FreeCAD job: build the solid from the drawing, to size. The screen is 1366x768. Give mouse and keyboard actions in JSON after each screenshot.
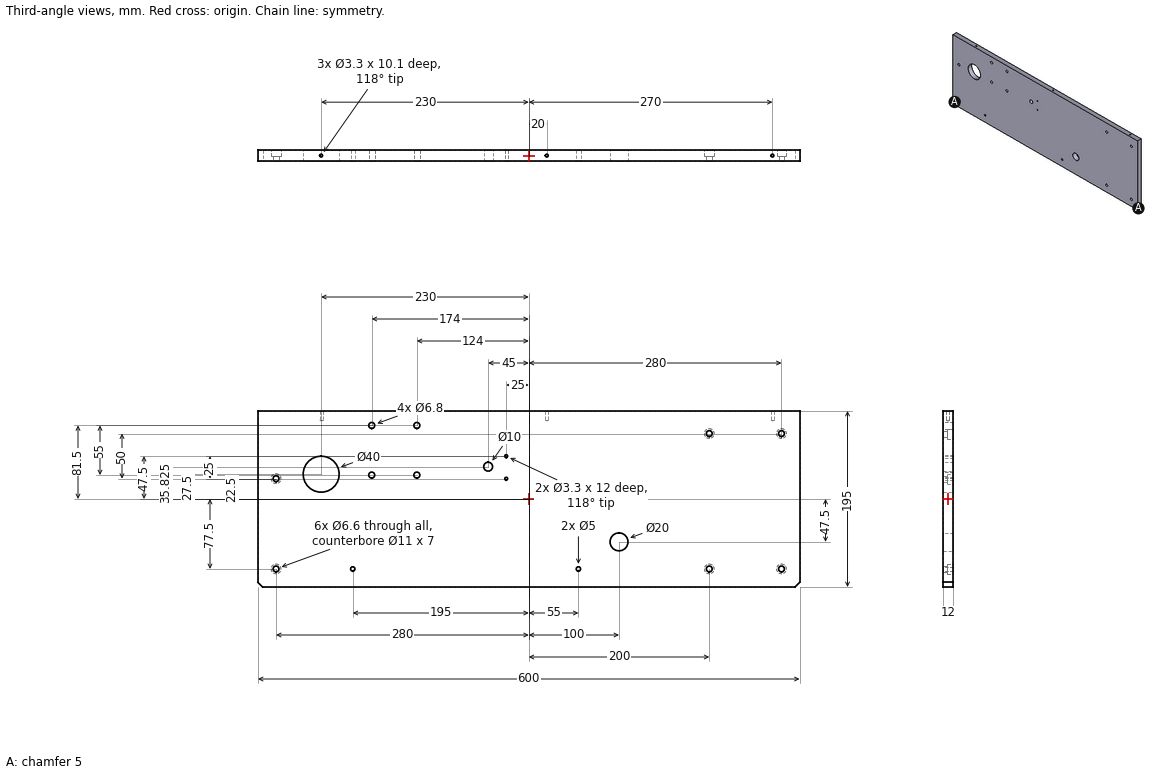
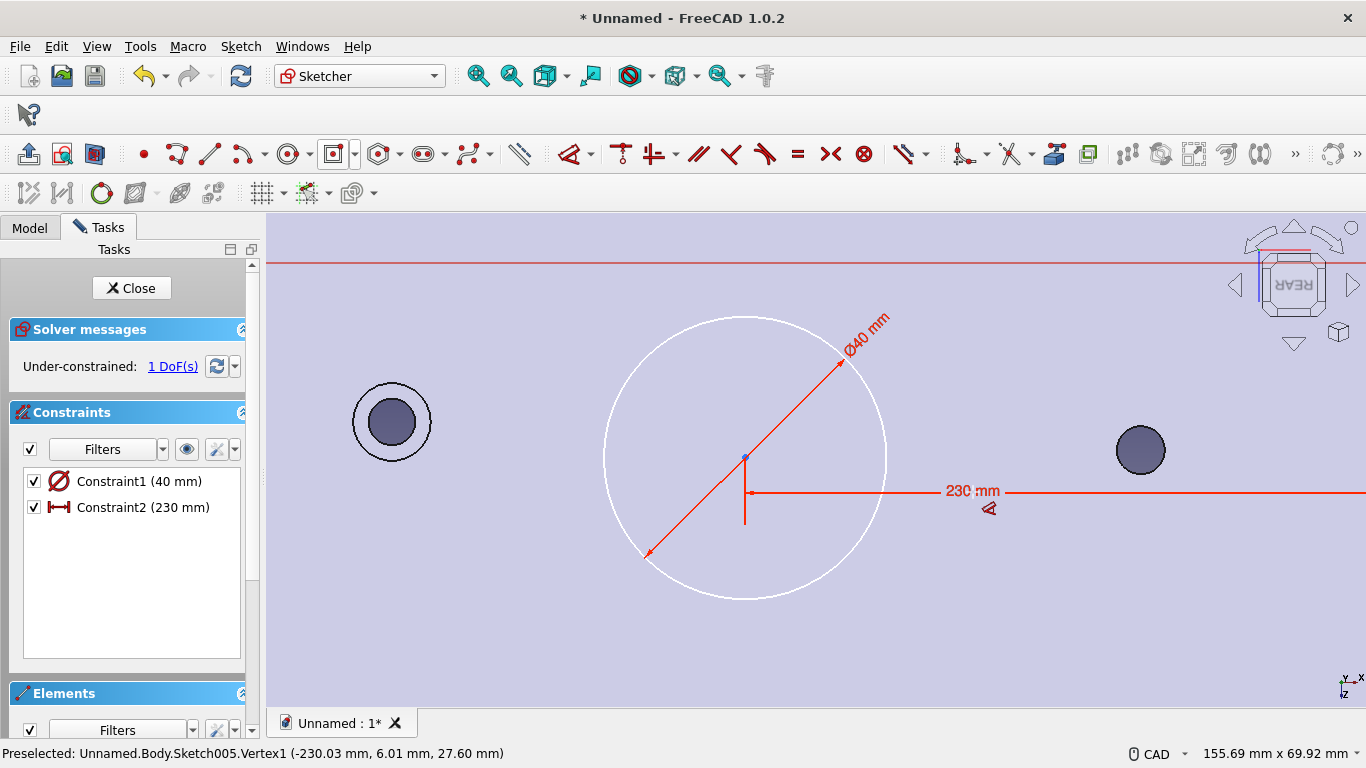
{"action": "left_click", "coordinate": [745, 458]}
{"action": "left_click", "coordinate": [711, 360]}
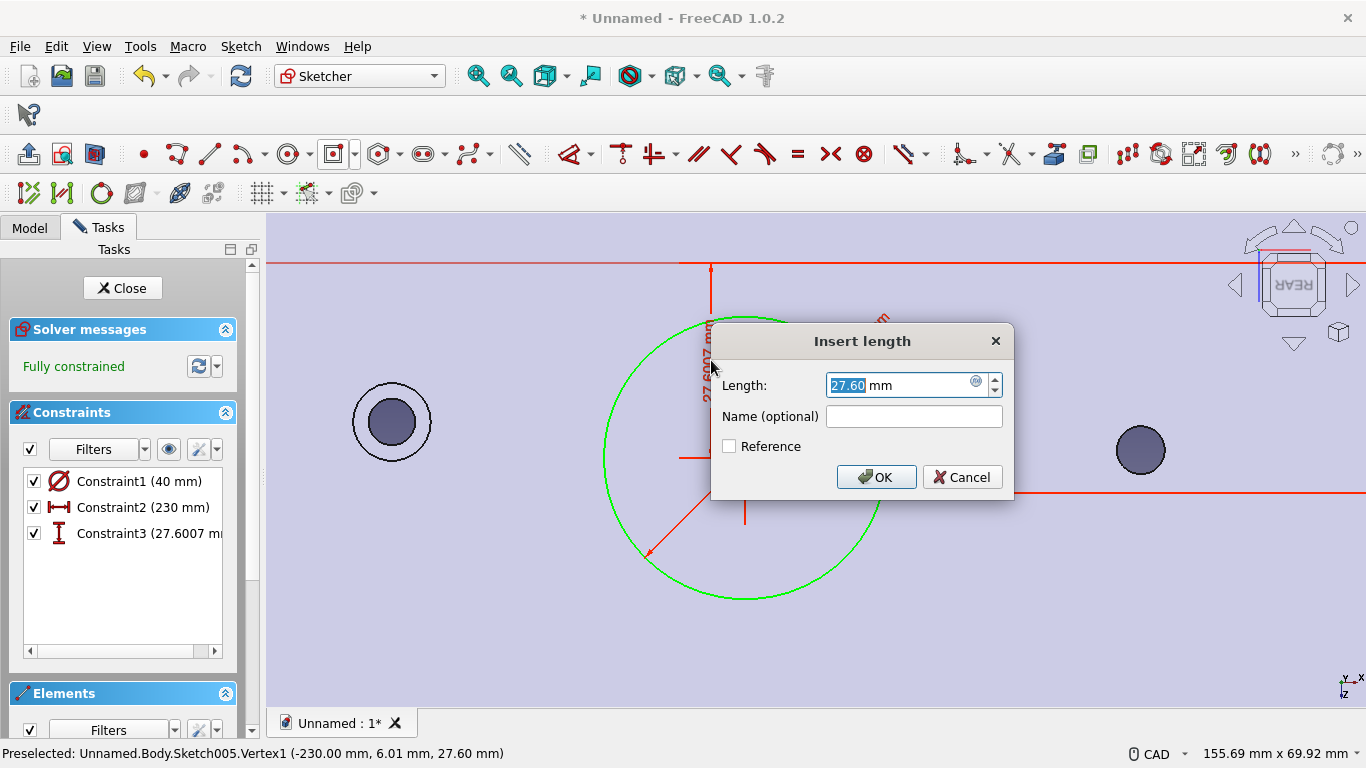
{"action": "type", "text": "27.5"}
{"action": "key", "text": "Return"}
{"action": "key", "text": "Escape"}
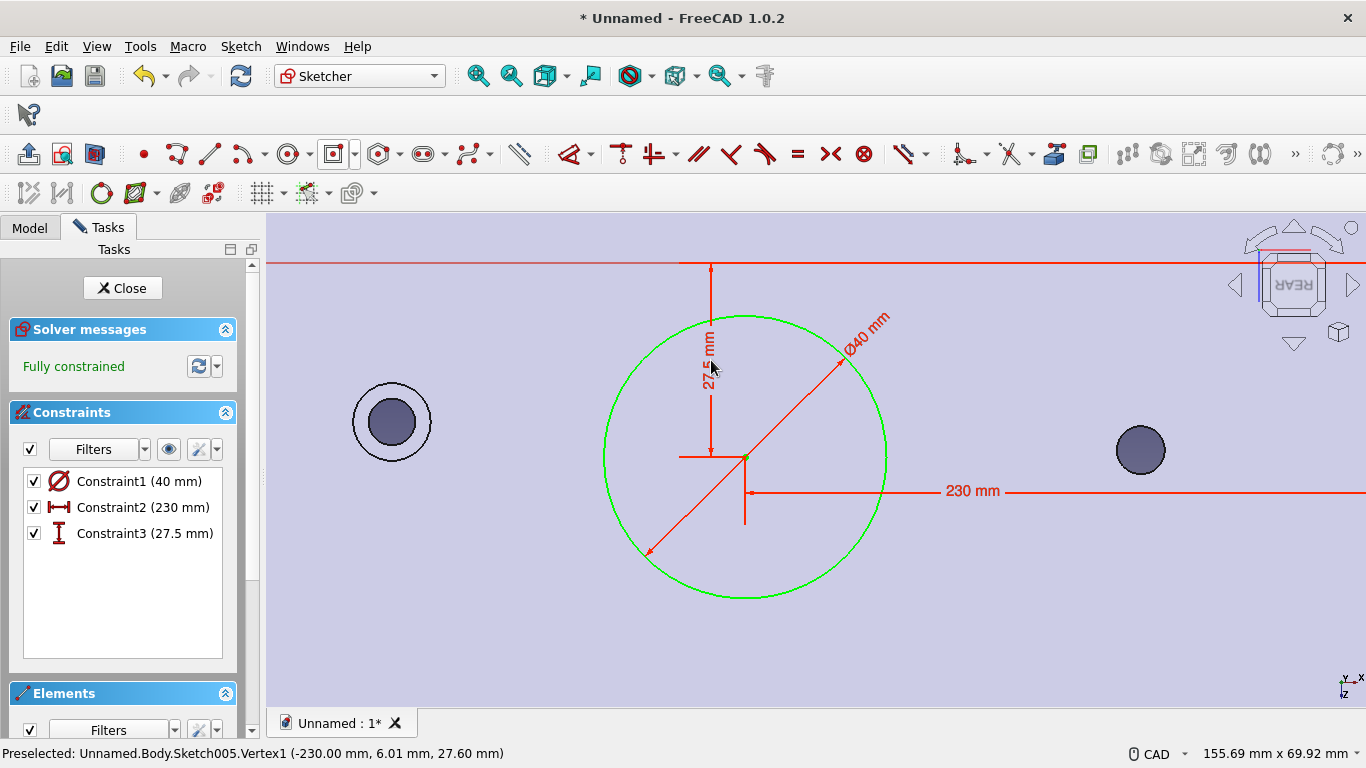
{"action": "left_click", "coordinate": [123, 288]}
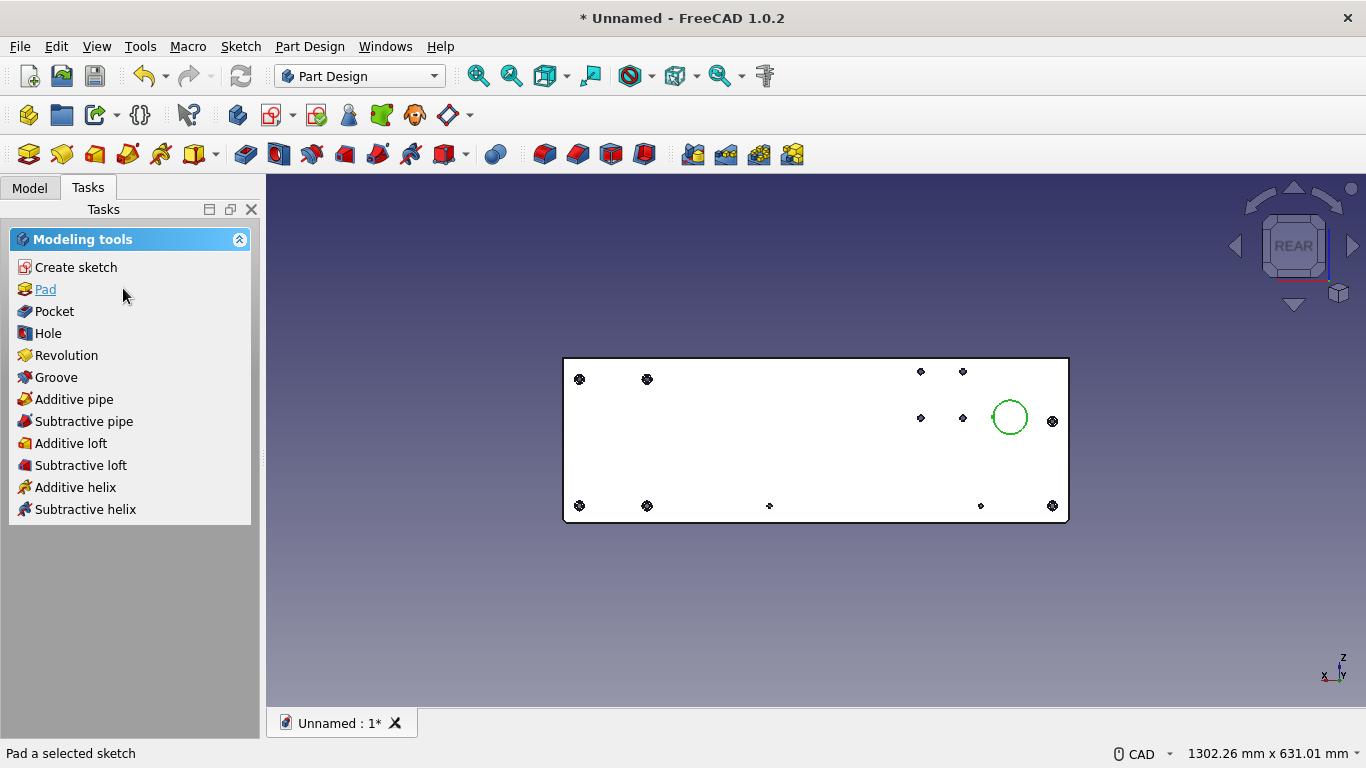
{"action": "left_click", "coordinate": [246, 154]}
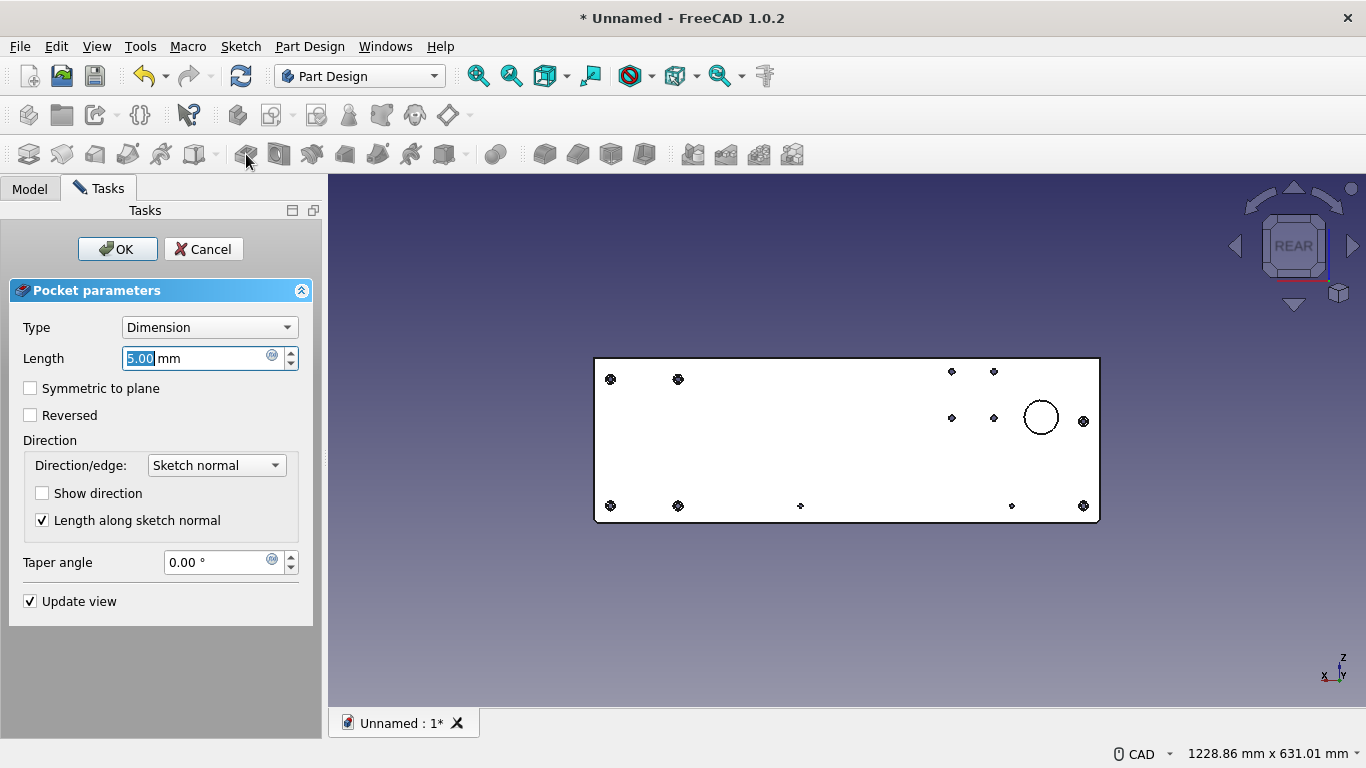
{"action": "left_click", "coordinate": [210, 328]}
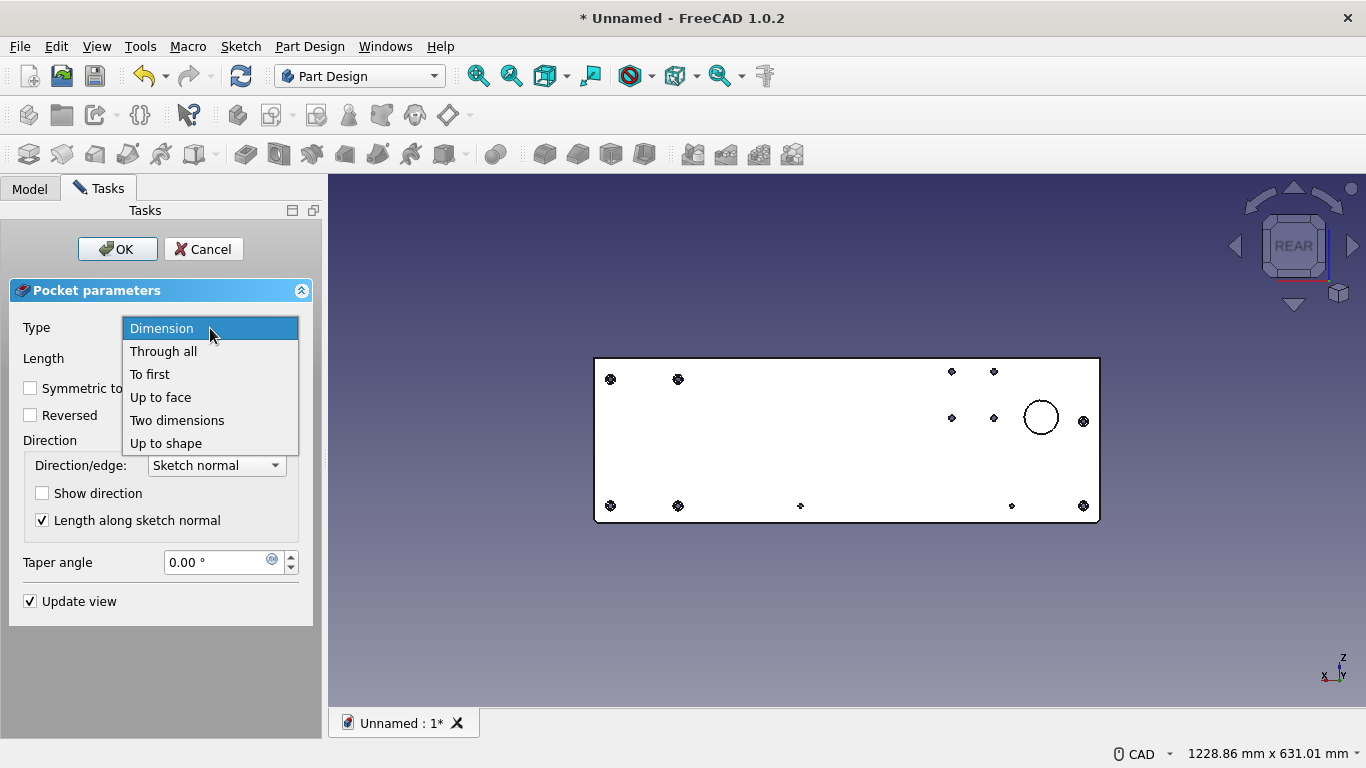
{"action": "left_click", "coordinate": [208, 352]}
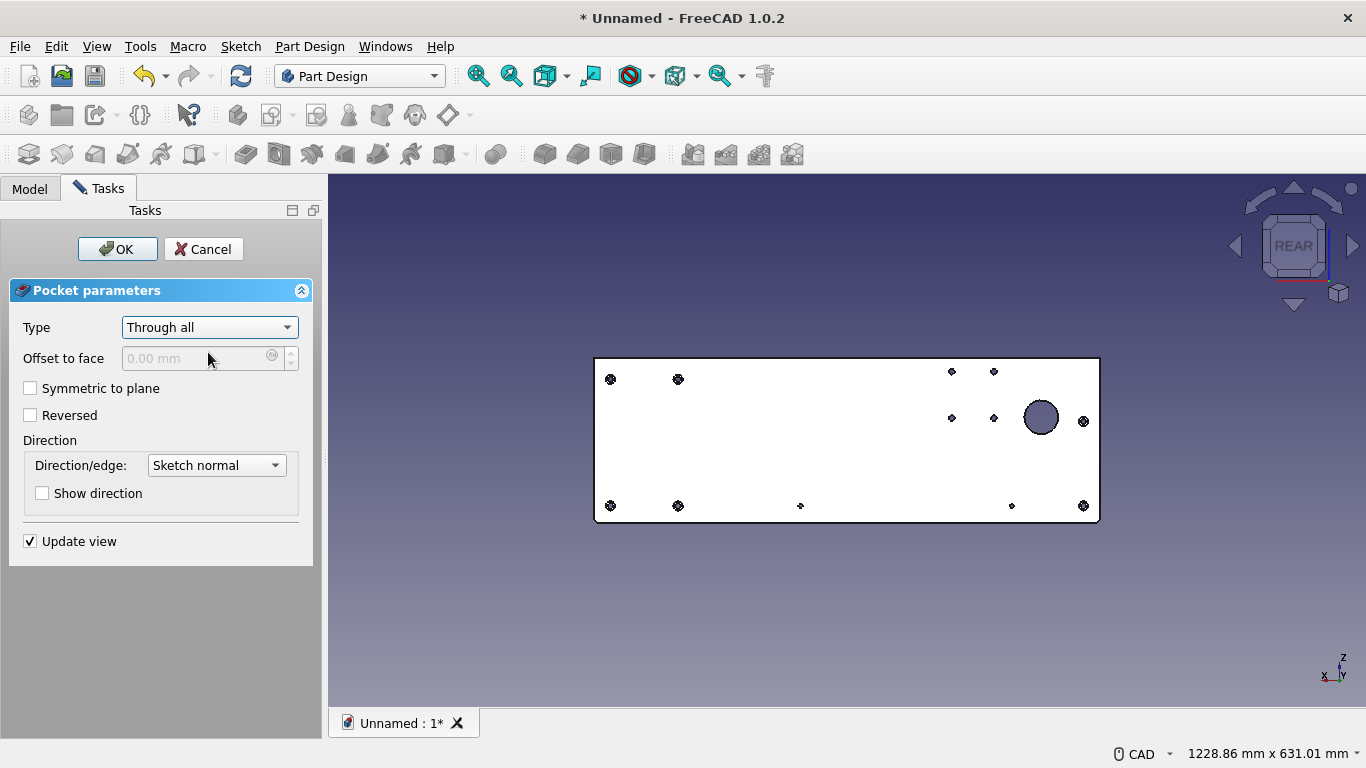
{"action": "left_click", "coordinate": [118, 249]}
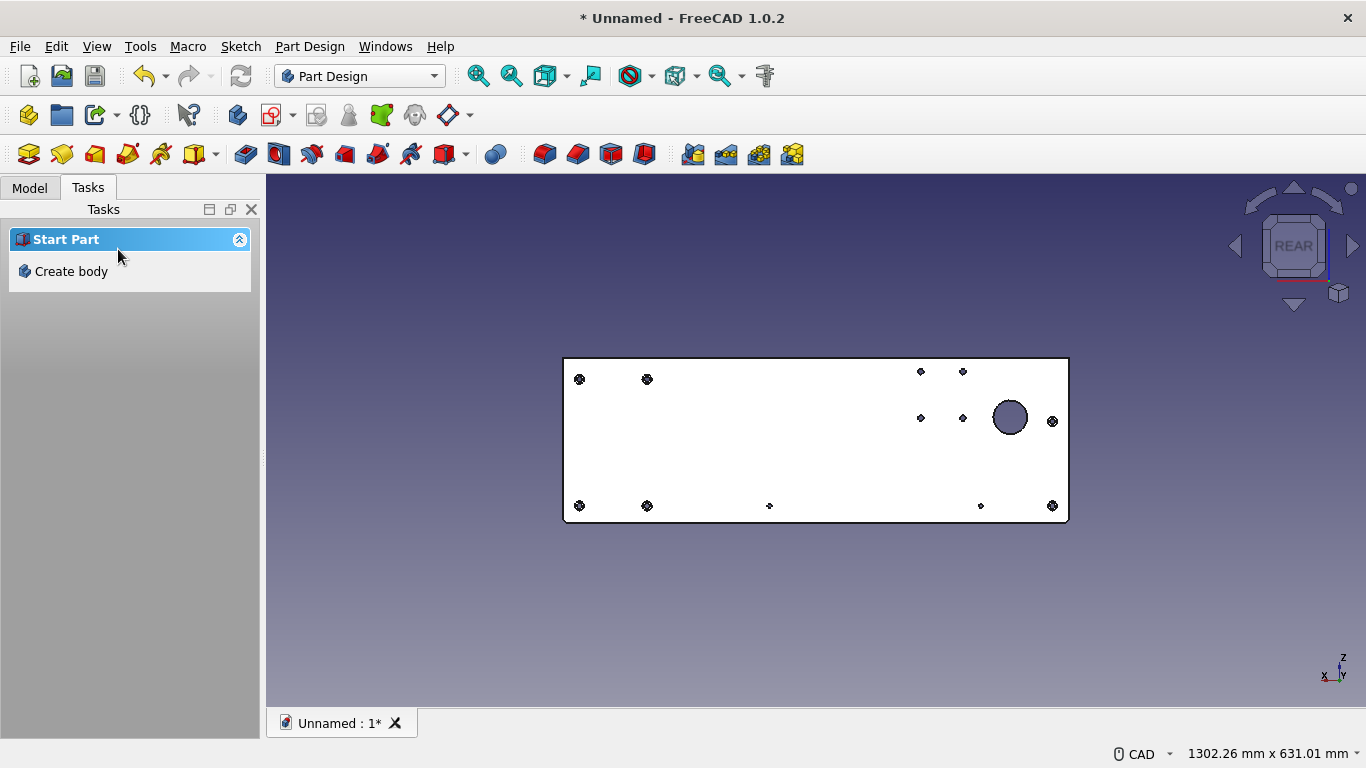
{"action": "left_click", "coordinate": [816, 439]}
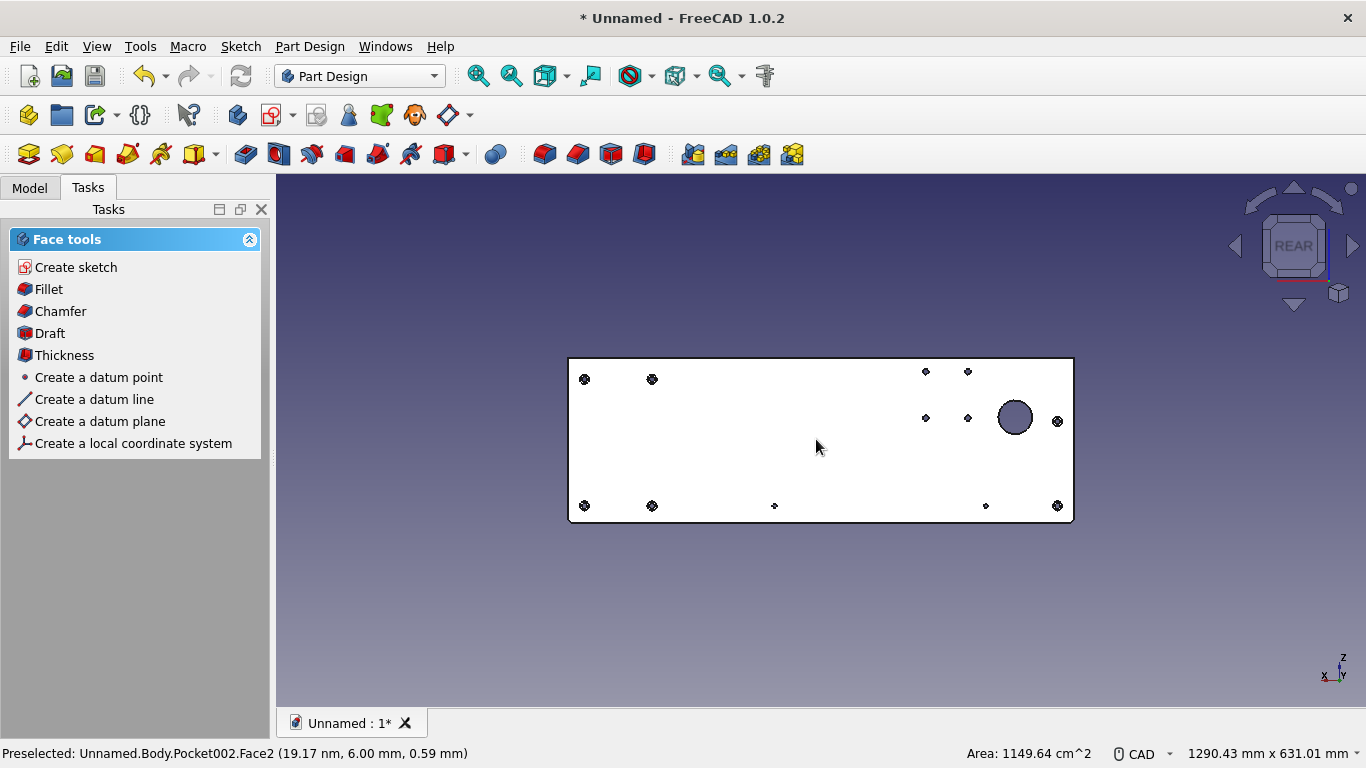
{"action": "left_click", "coordinate": [270, 116]}